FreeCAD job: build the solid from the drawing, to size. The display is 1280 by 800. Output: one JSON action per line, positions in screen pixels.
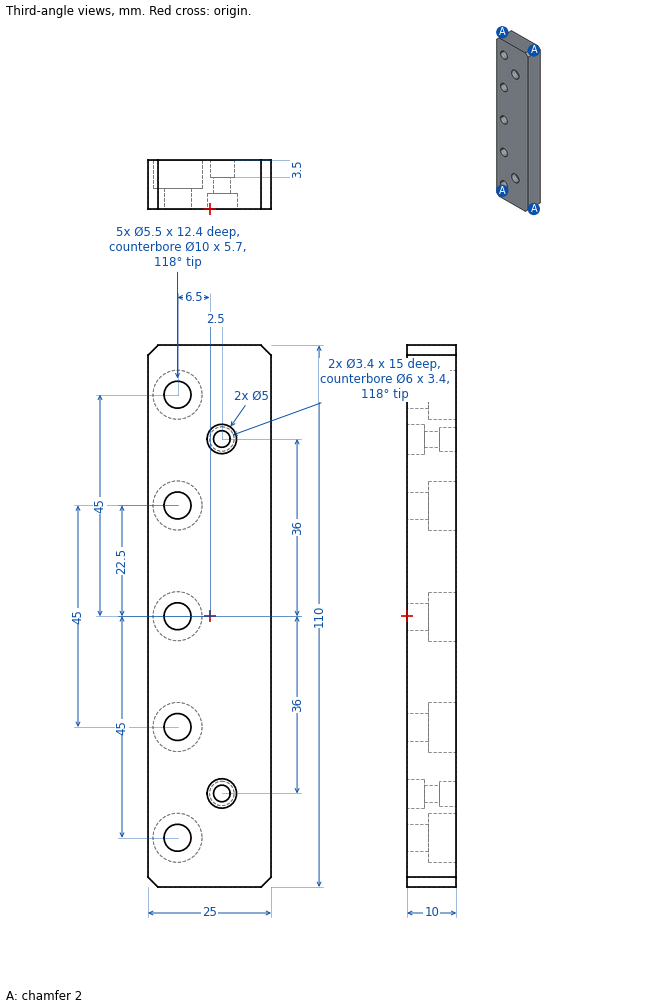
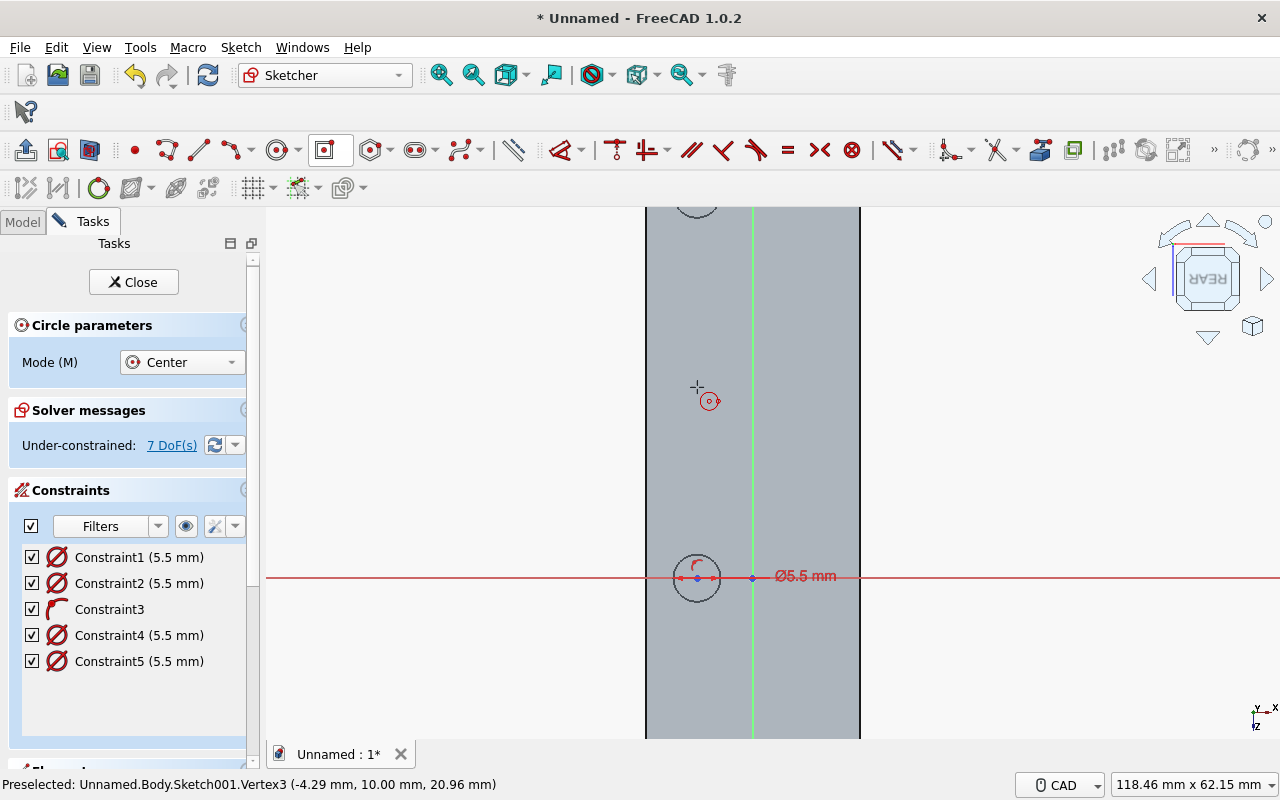
{"action": "left_click", "coordinate": [697, 386]}
{"action": "mouse_move", "coordinate": [714, 369]}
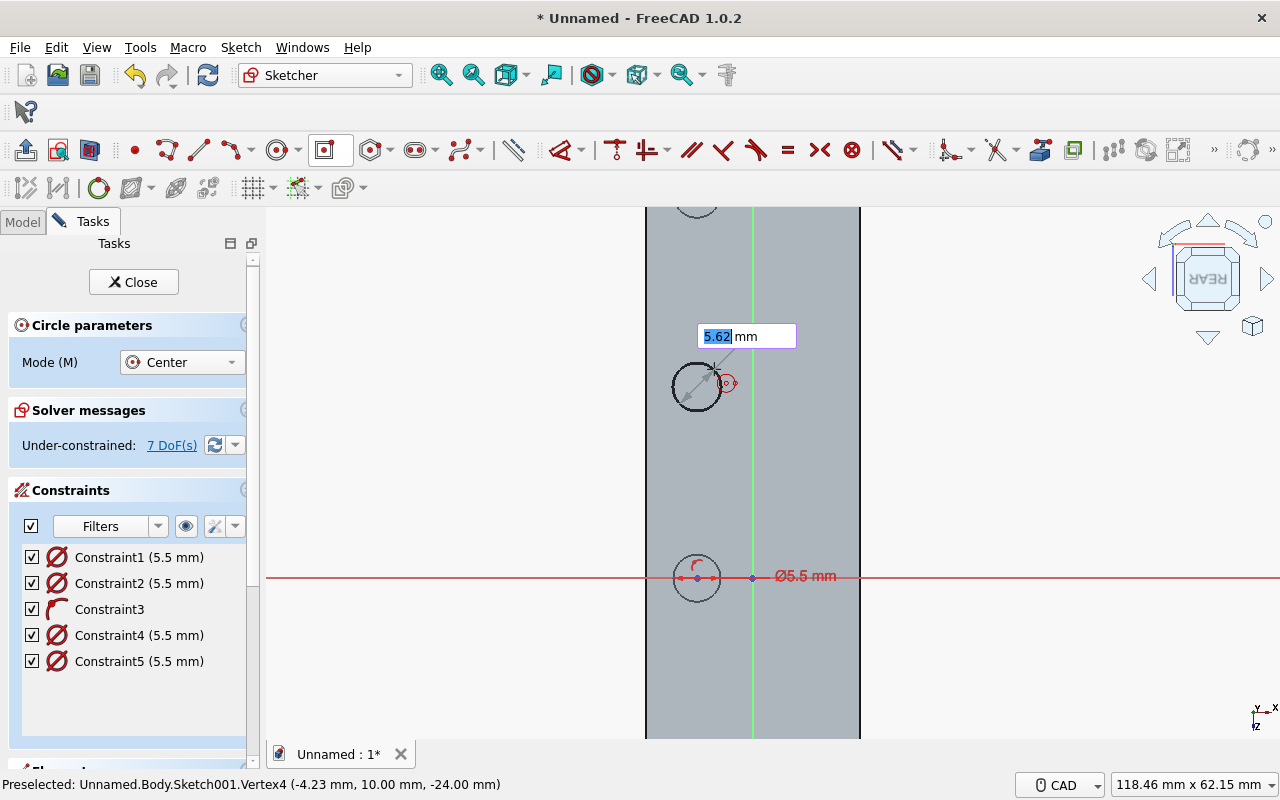
{"action": "type", "text": "5.5"}
{"action": "key", "text": "Return"}
{"action": "key", "text": "Escape"}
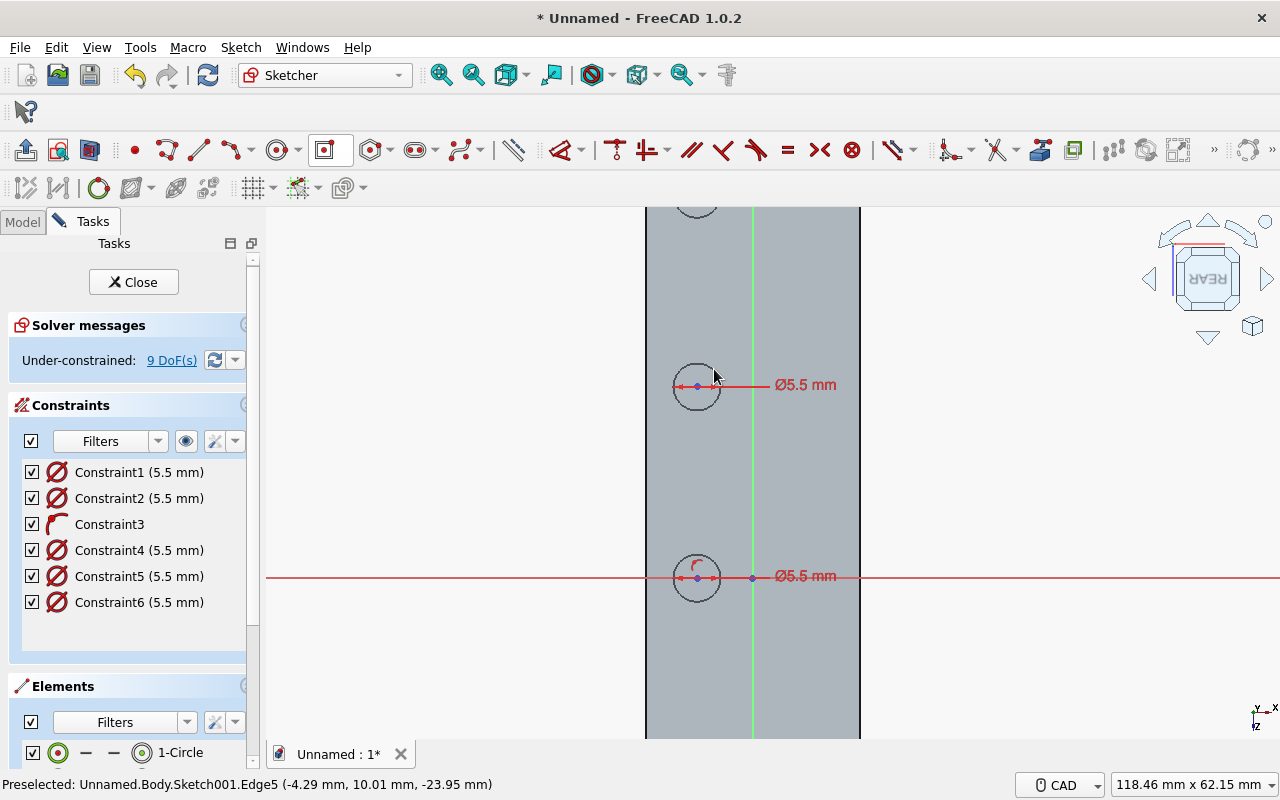
{"action": "scroll", "coordinate": [697, 387], "scroll_direction": "down", "scroll_amount": 4}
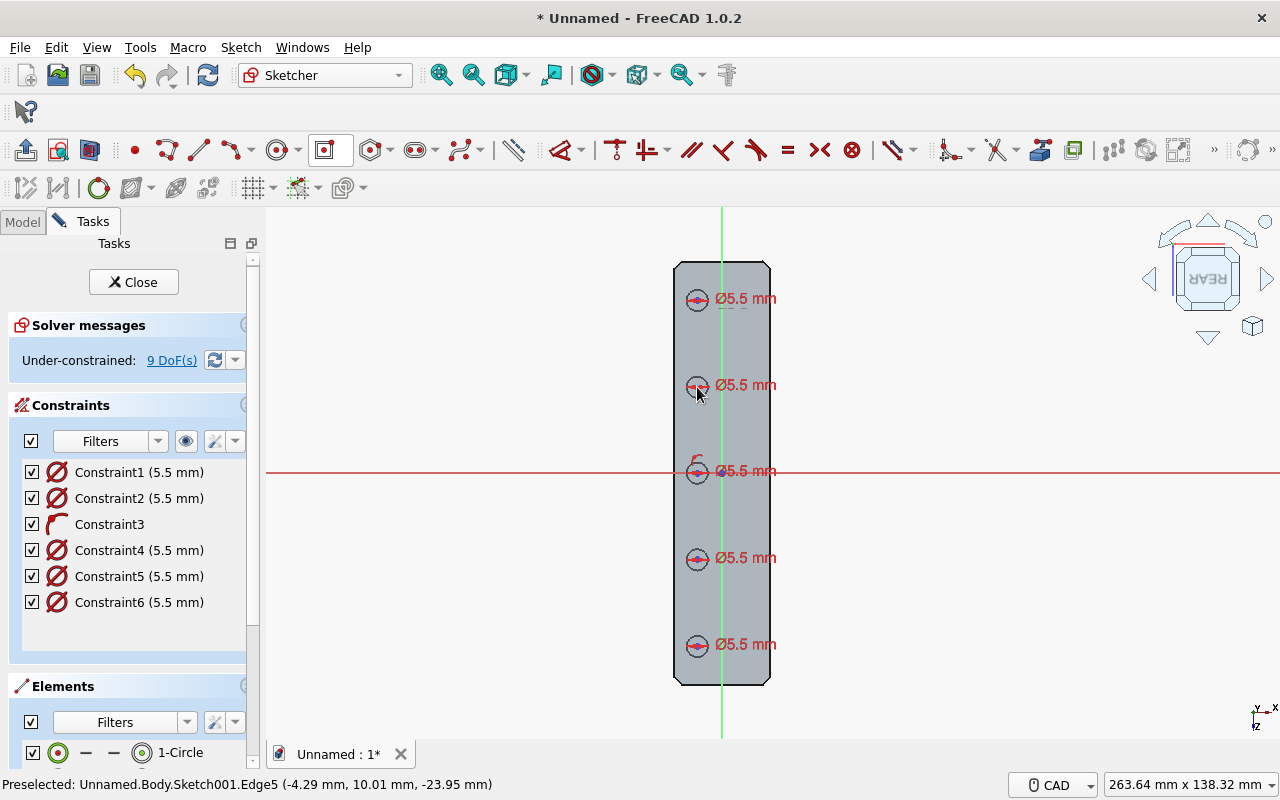
{"action": "left_click", "coordinate": [697, 646]}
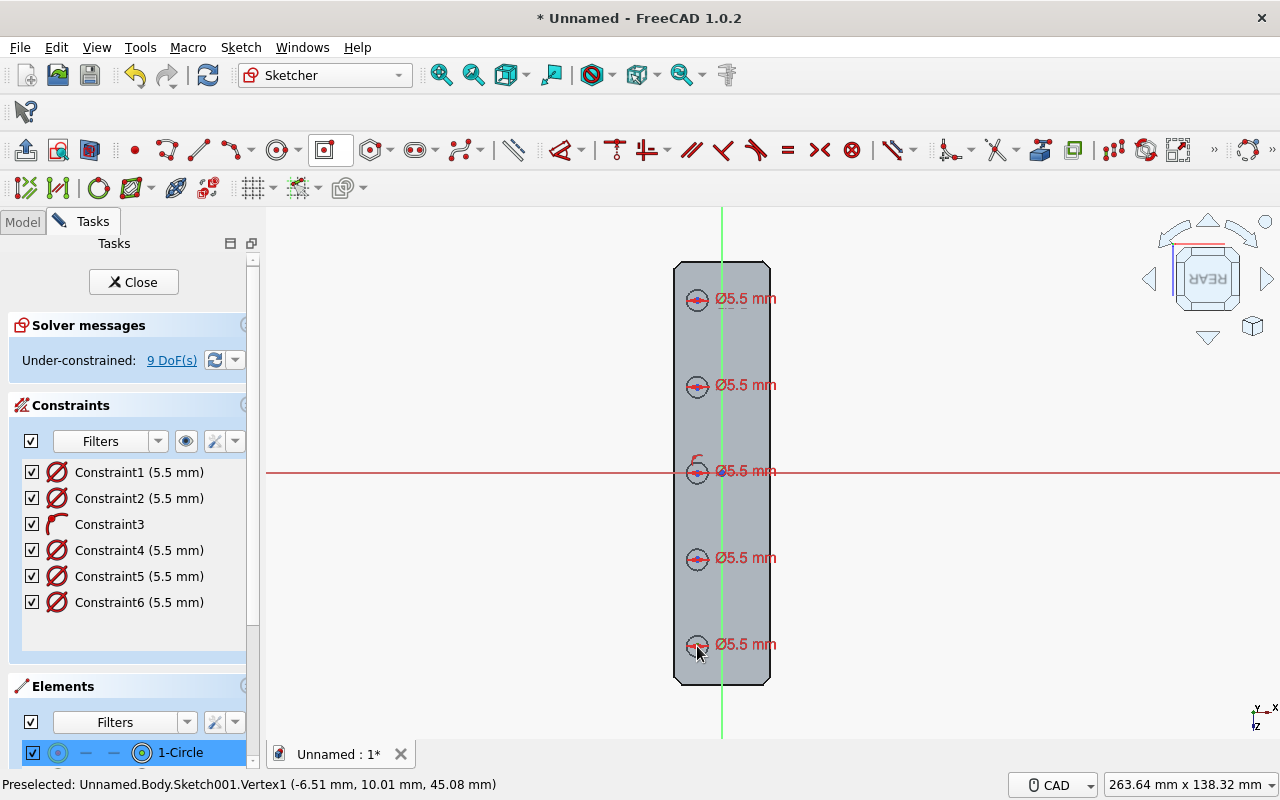
{"action": "left_click", "coordinate": [697, 473]}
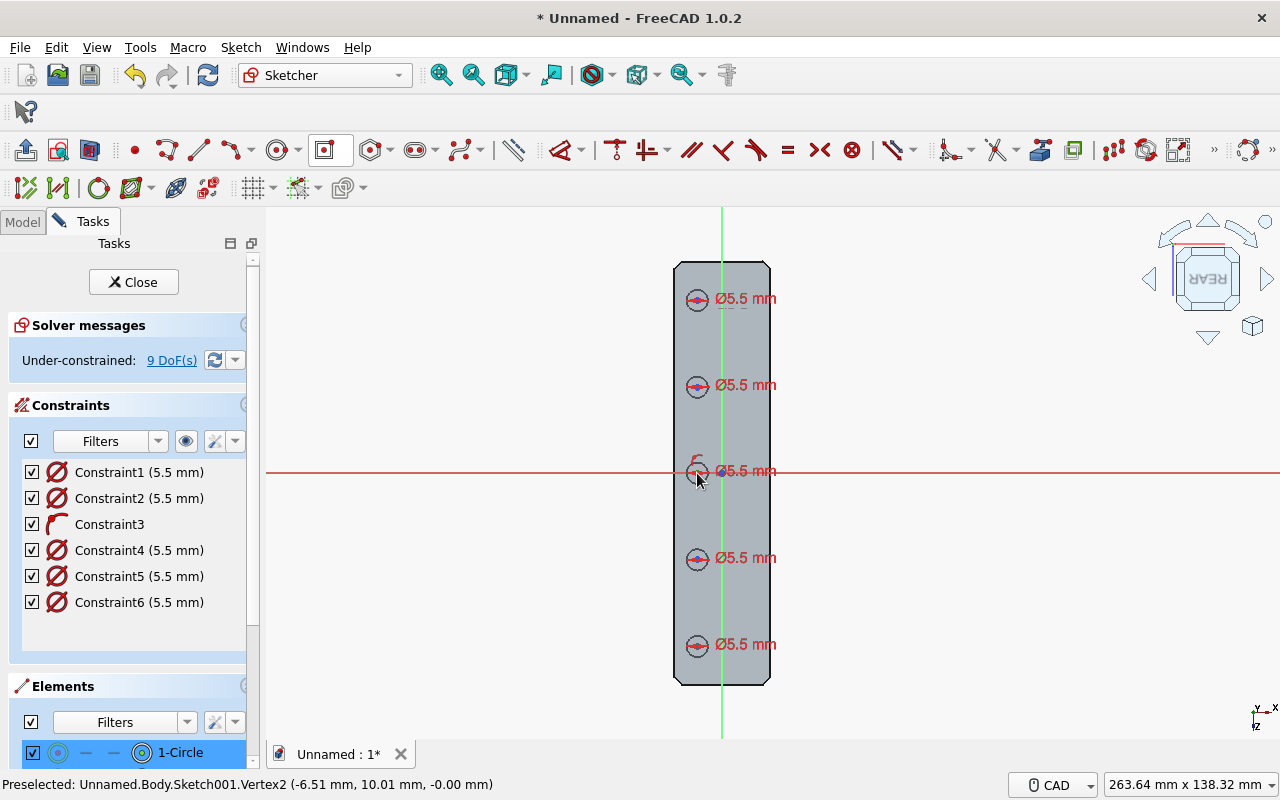
{"action": "left_click", "coordinate": [670, 150]}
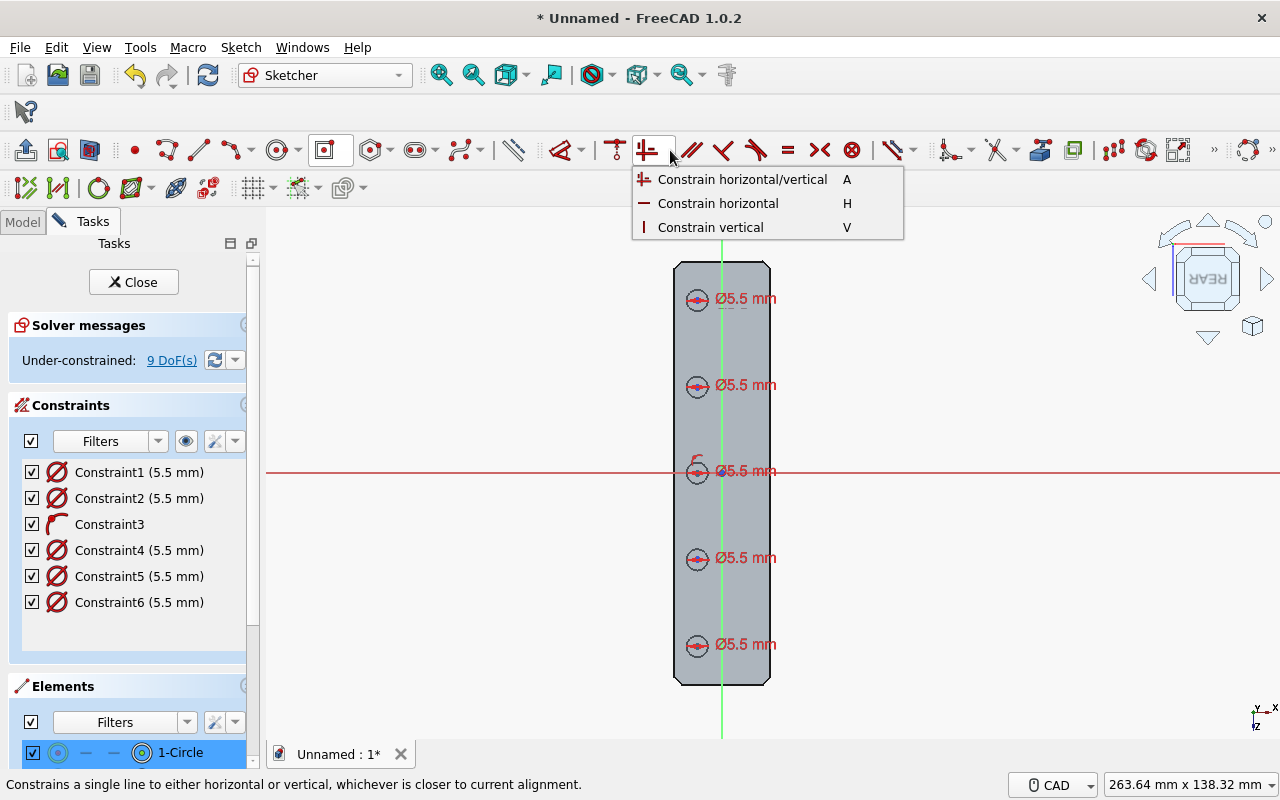
{"action": "left_click", "coordinate": [768, 227]}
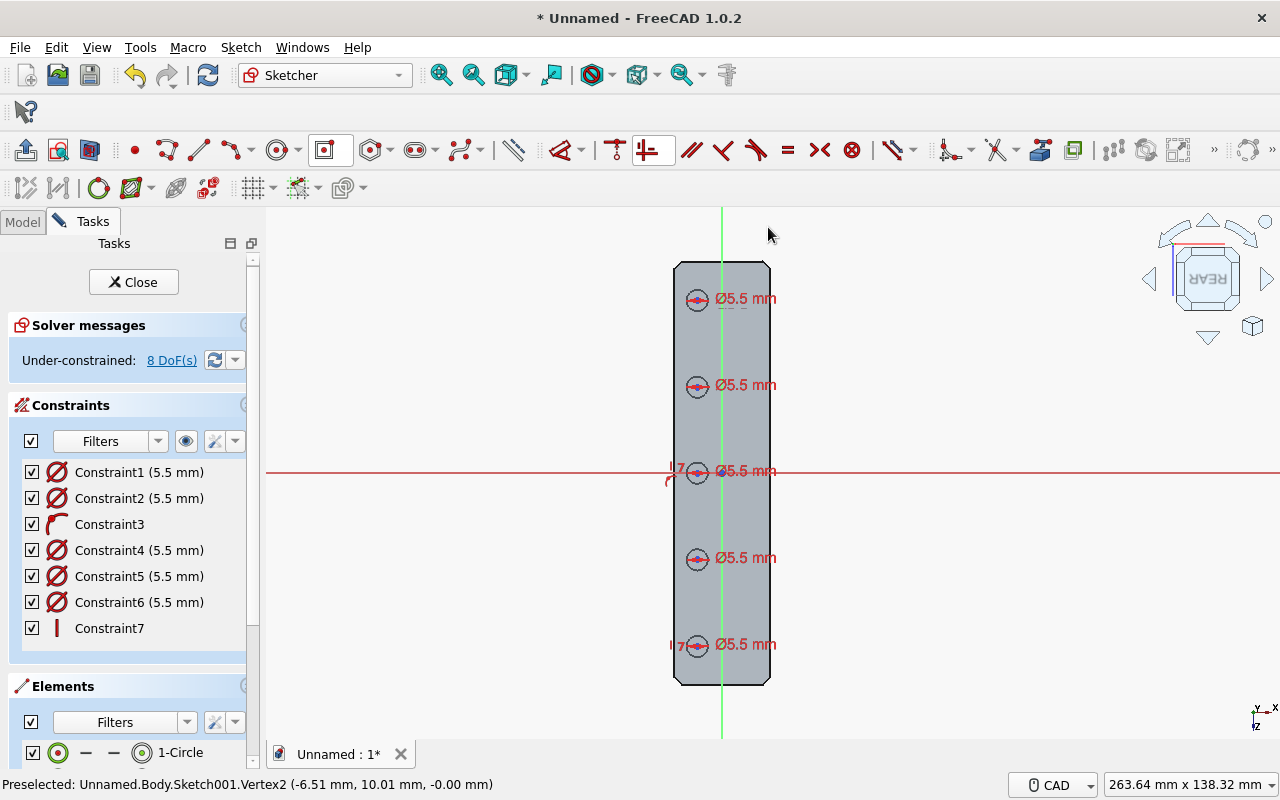
{"action": "left_click", "coordinate": [697, 473]}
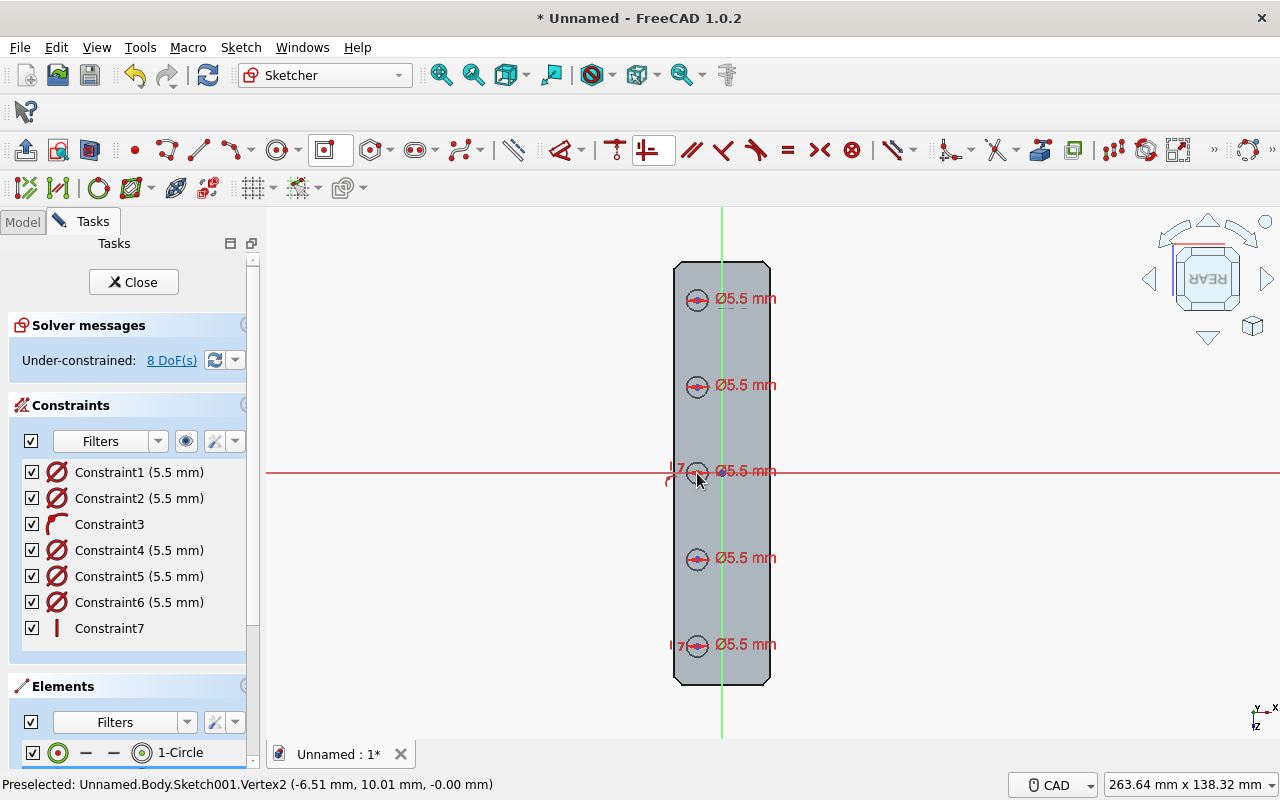
{"action": "left_click", "coordinate": [697, 301]}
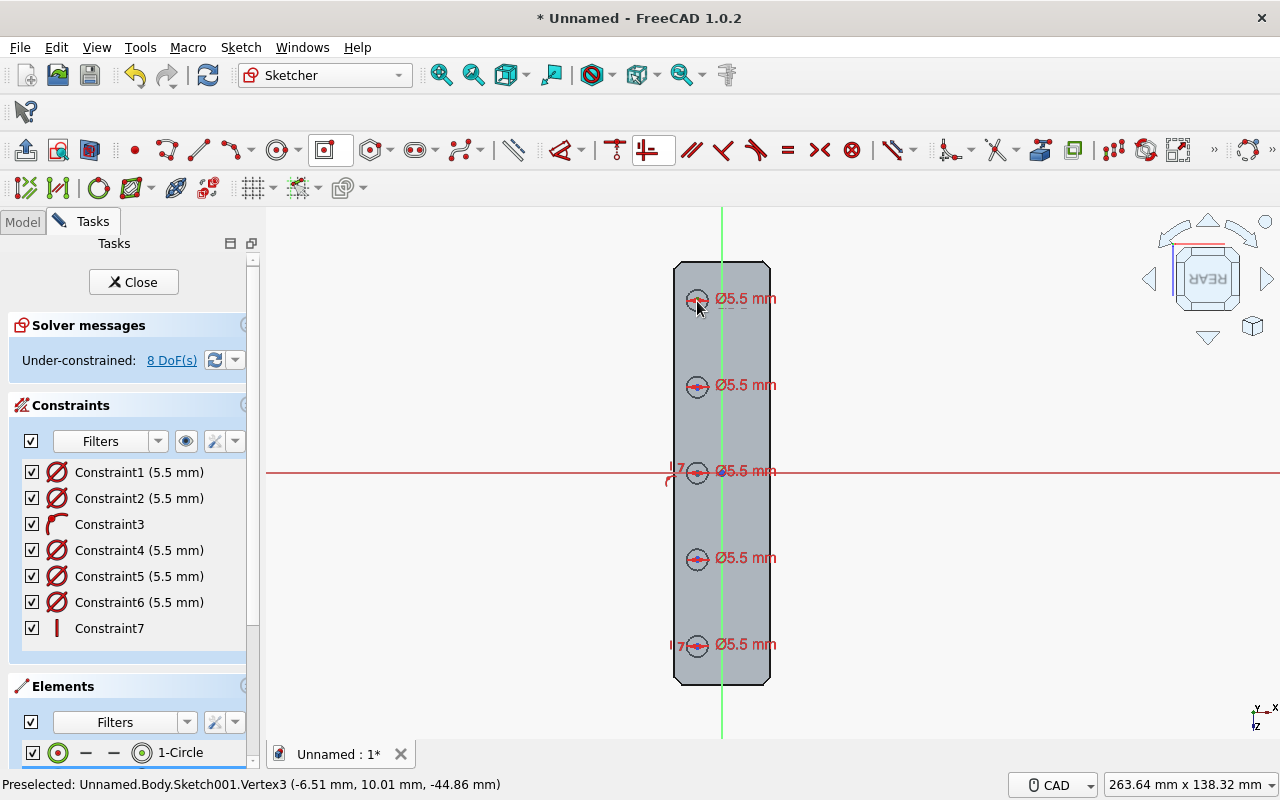
{"action": "key", "text": "v"}